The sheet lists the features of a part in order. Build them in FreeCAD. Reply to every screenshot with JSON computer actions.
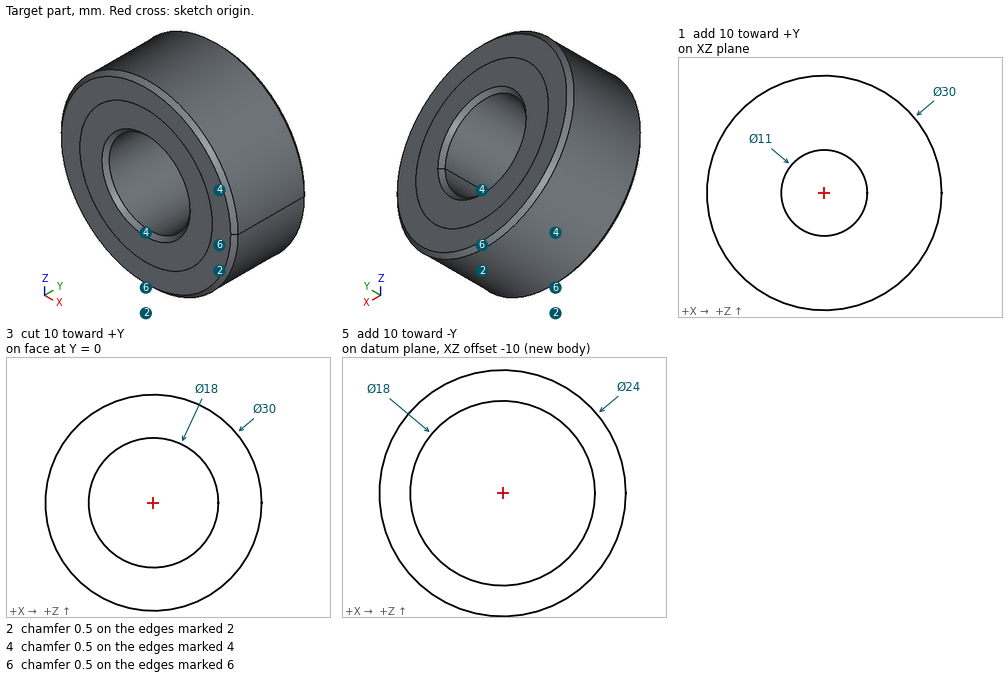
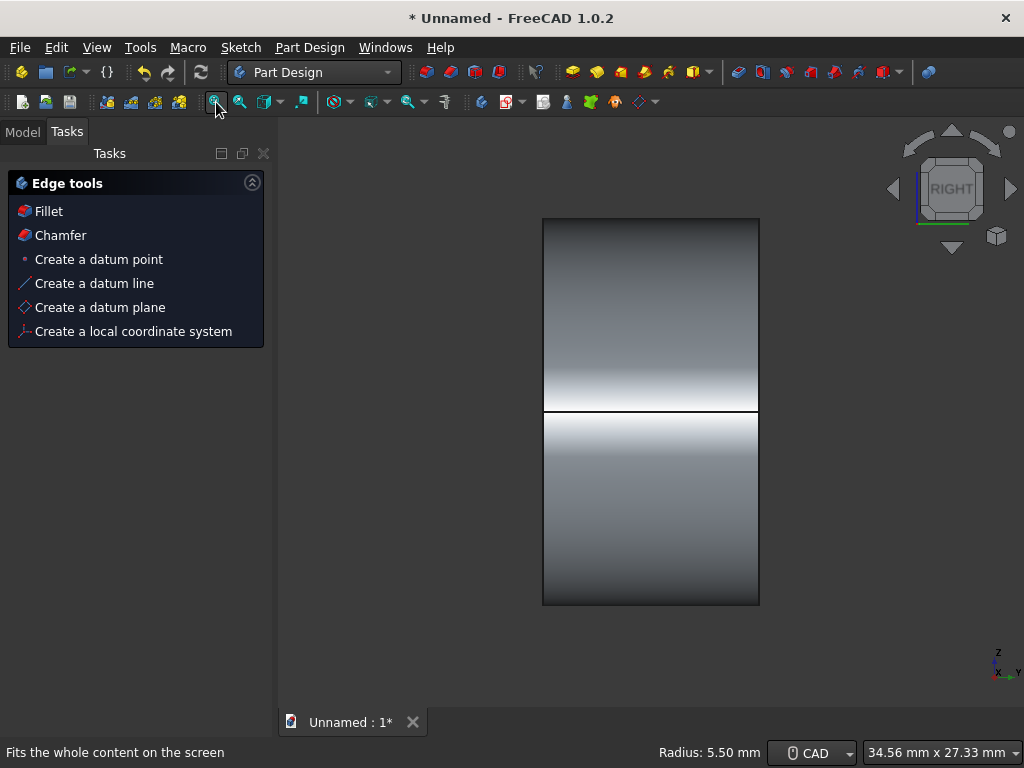
{"action": "key", "text": "5"}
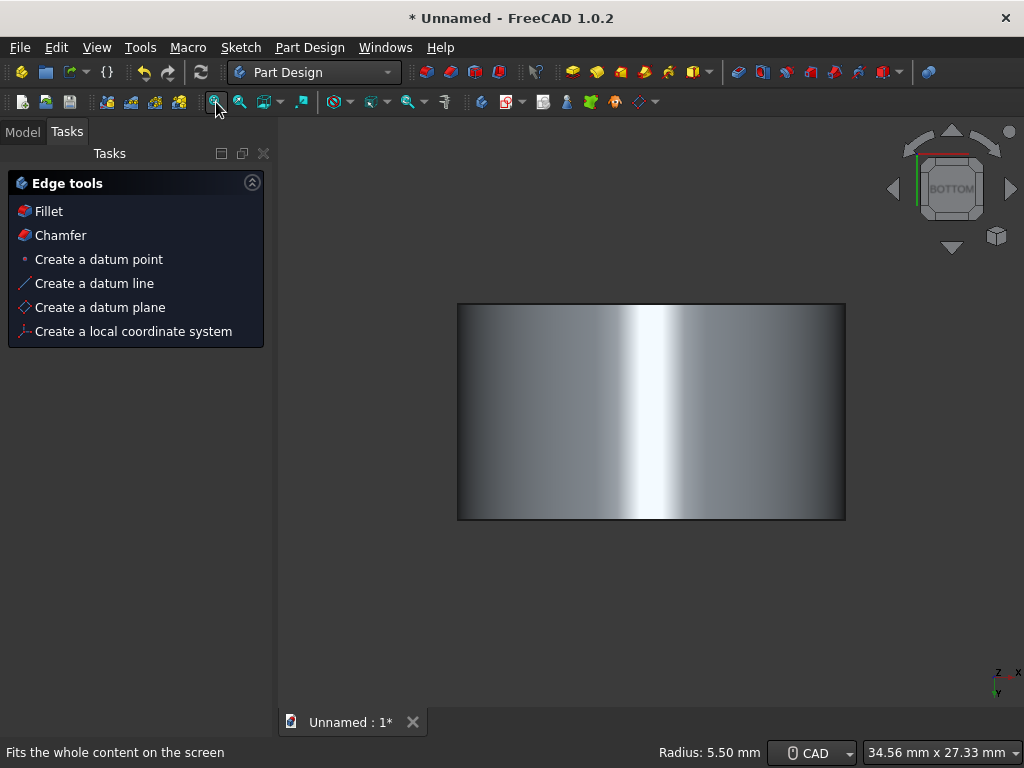
{"action": "key", "text": "4"}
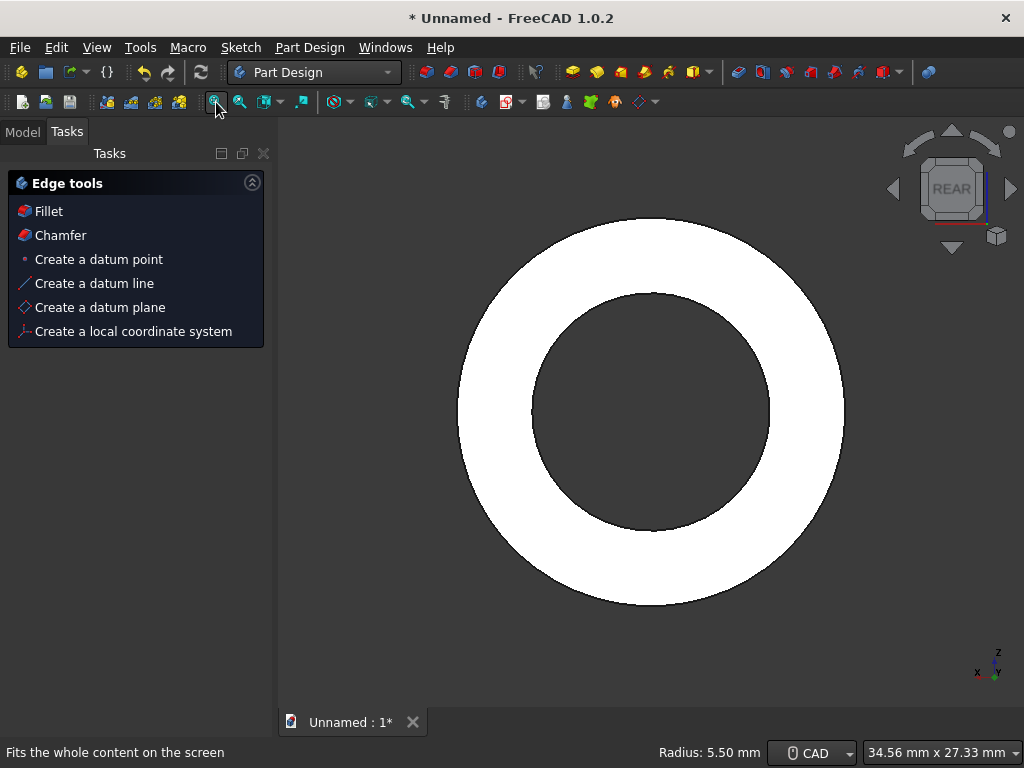
{"action": "left_click", "coordinate": [770, 411], "text": "ctrl"}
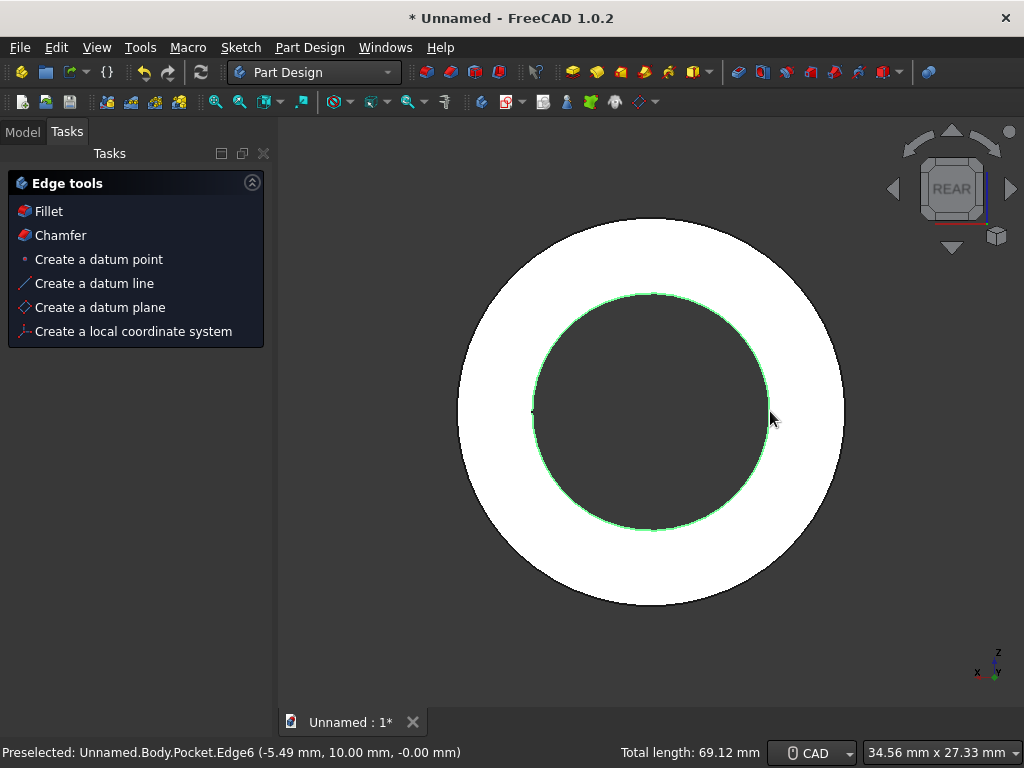
{"action": "left_click", "coordinate": [452, 72]}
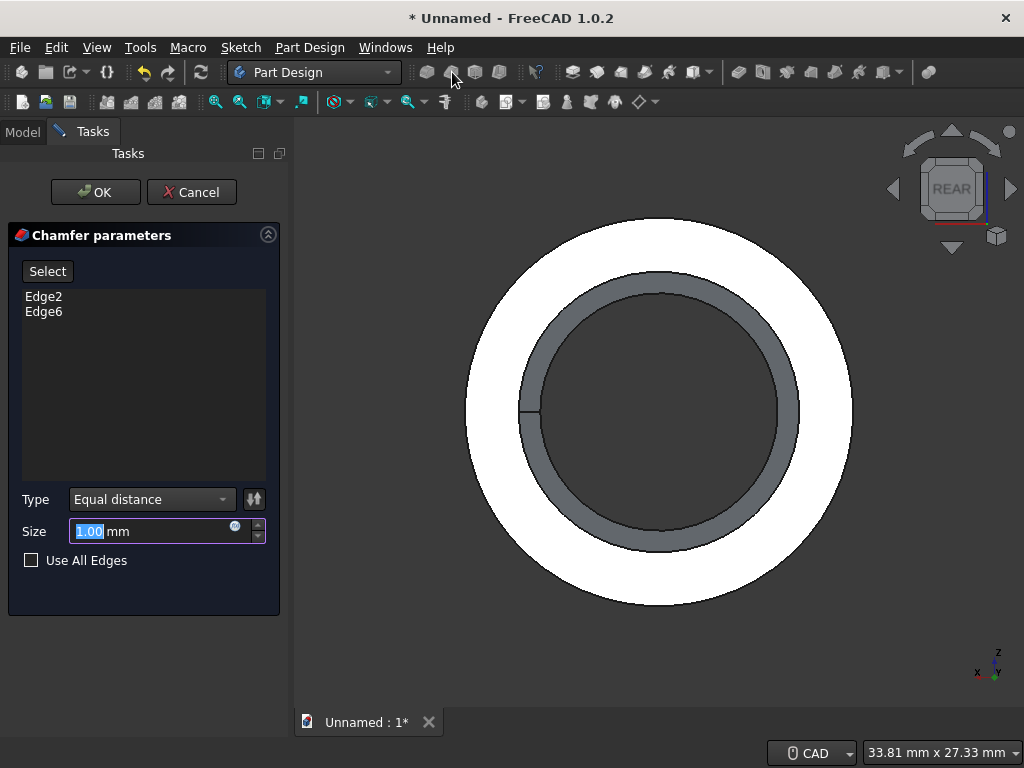
{"action": "type", "text": "0.5"}
{"action": "key", "text": "Tab"}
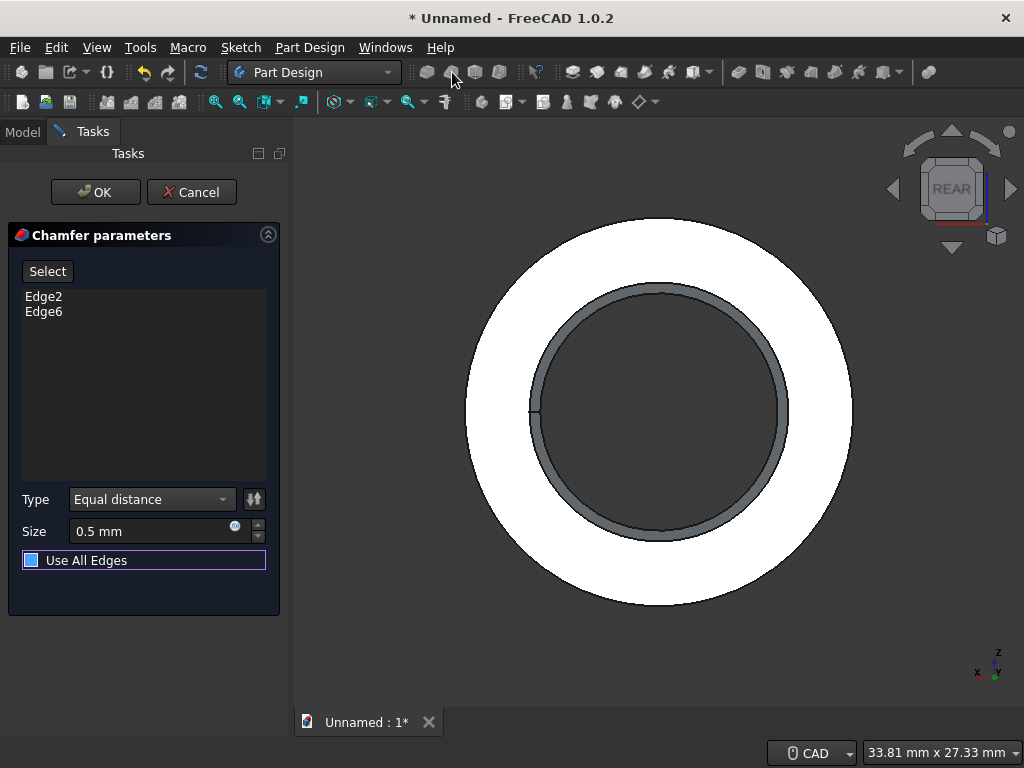
{"action": "left_click", "coordinate": [96, 192]}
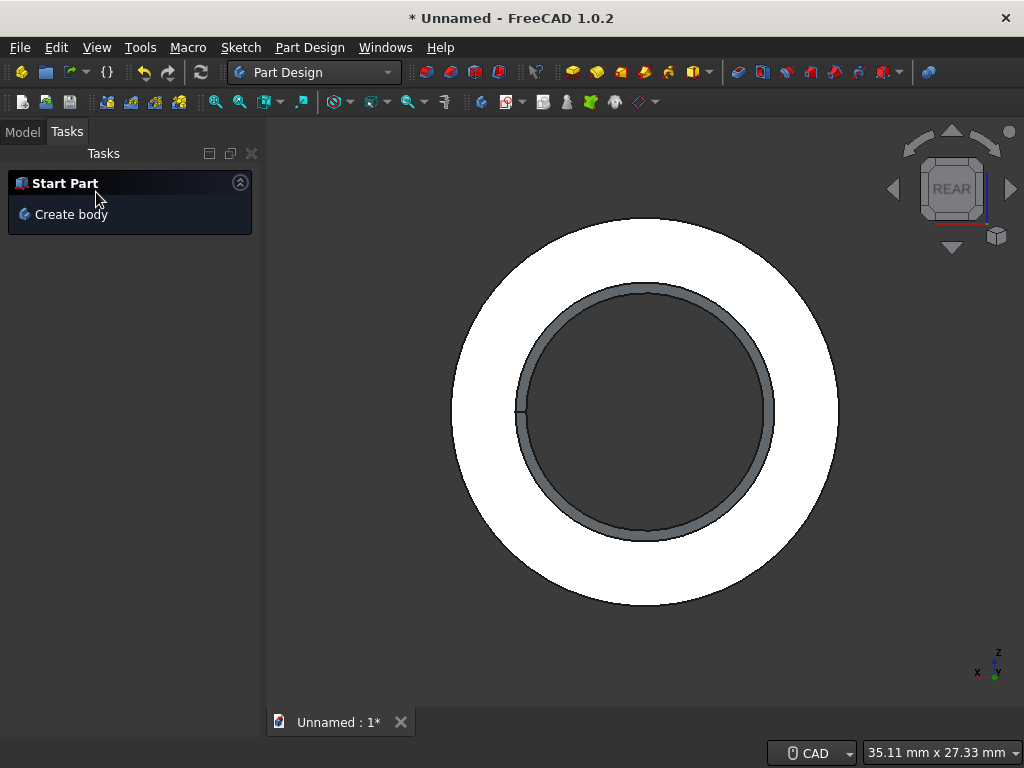
{"action": "left_click", "coordinate": [482, 102]}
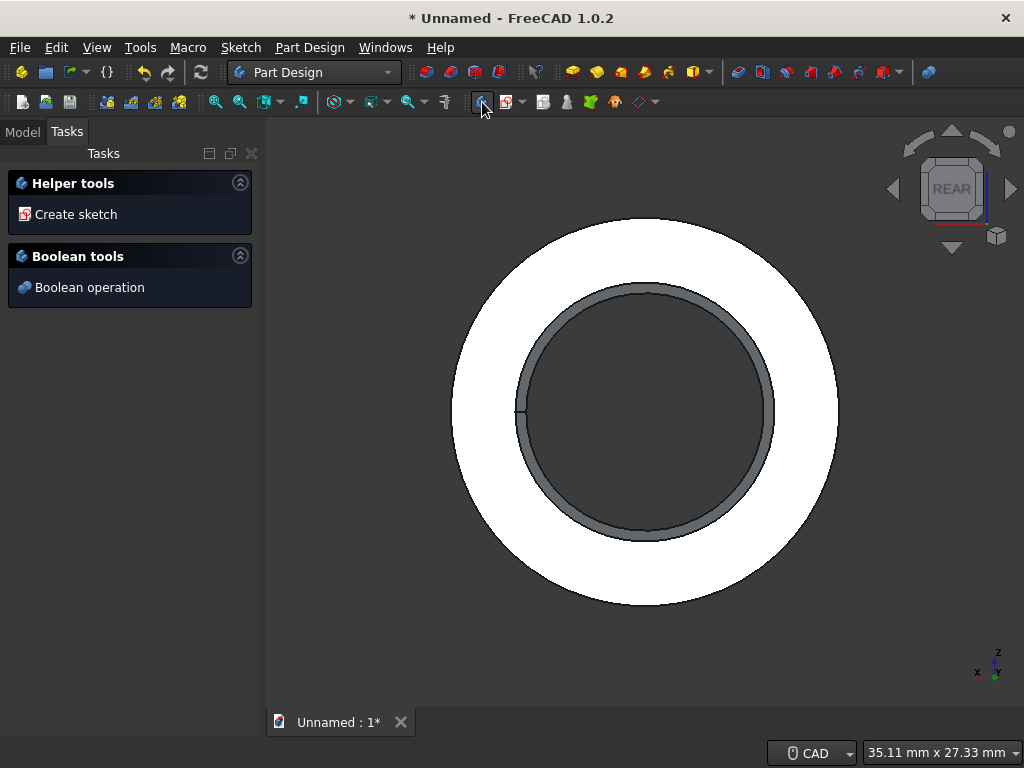
{"action": "left_click", "coordinate": [23, 131]}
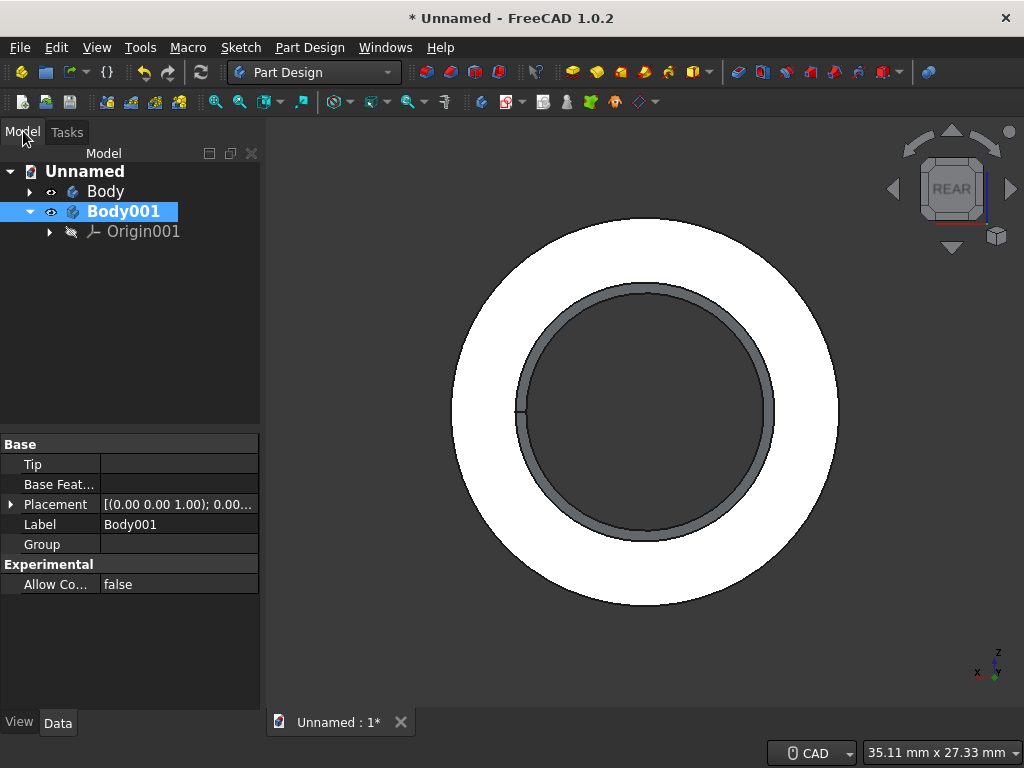
{"action": "left_click", "coordinate": [50, 232]}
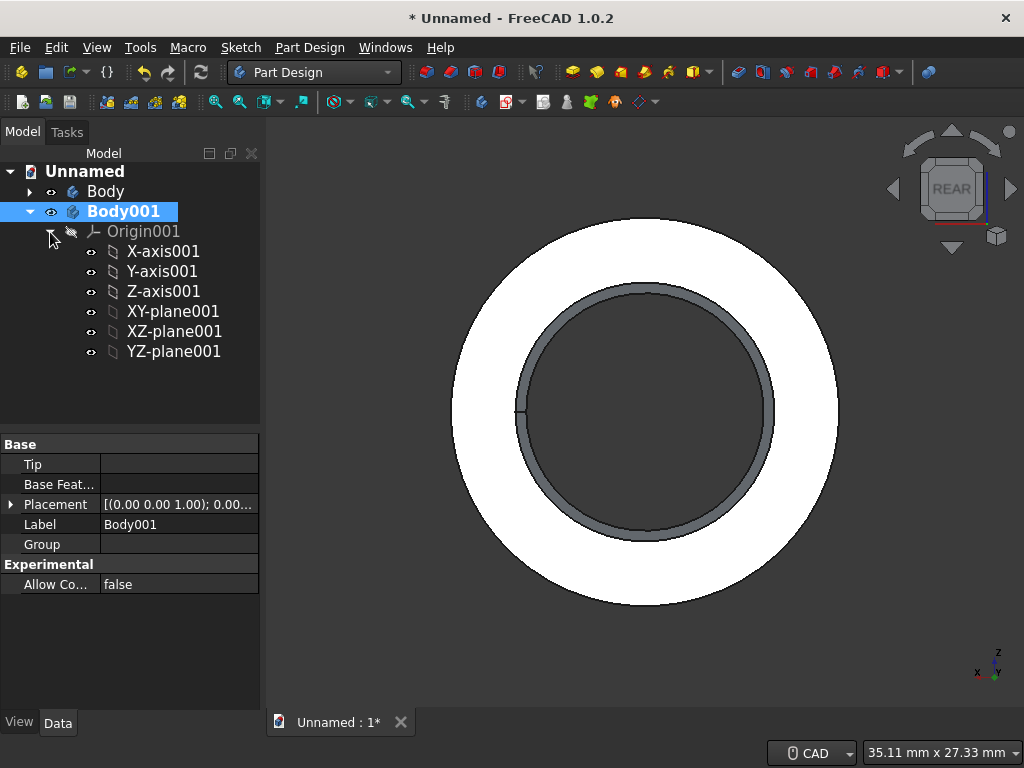
{"action": "left_click", "coordinate": [136, 332]}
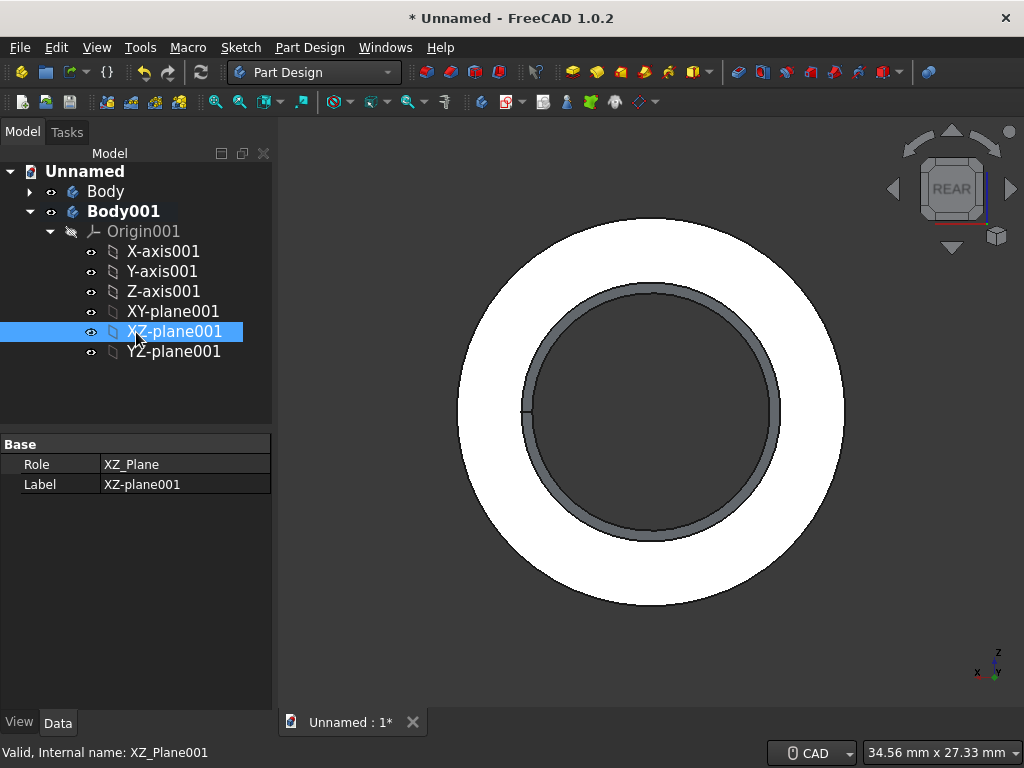
{"action": "left_click", "coordinate": [640, 102]}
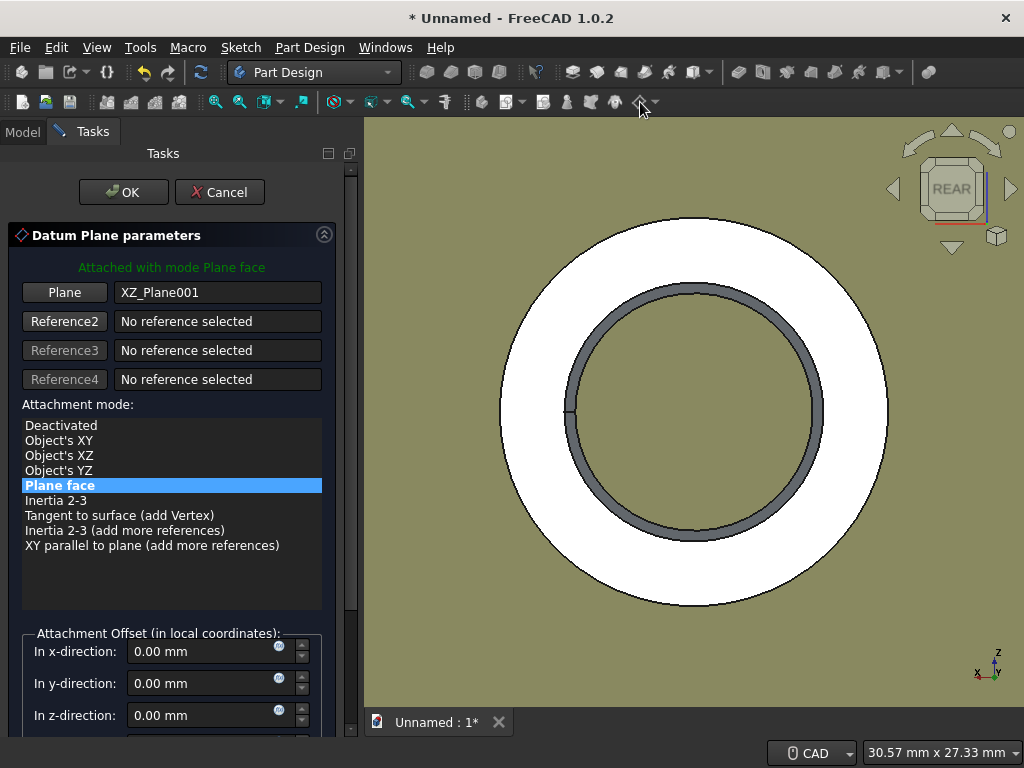
{"action": "triple_click", "coordinate": [210, 715]}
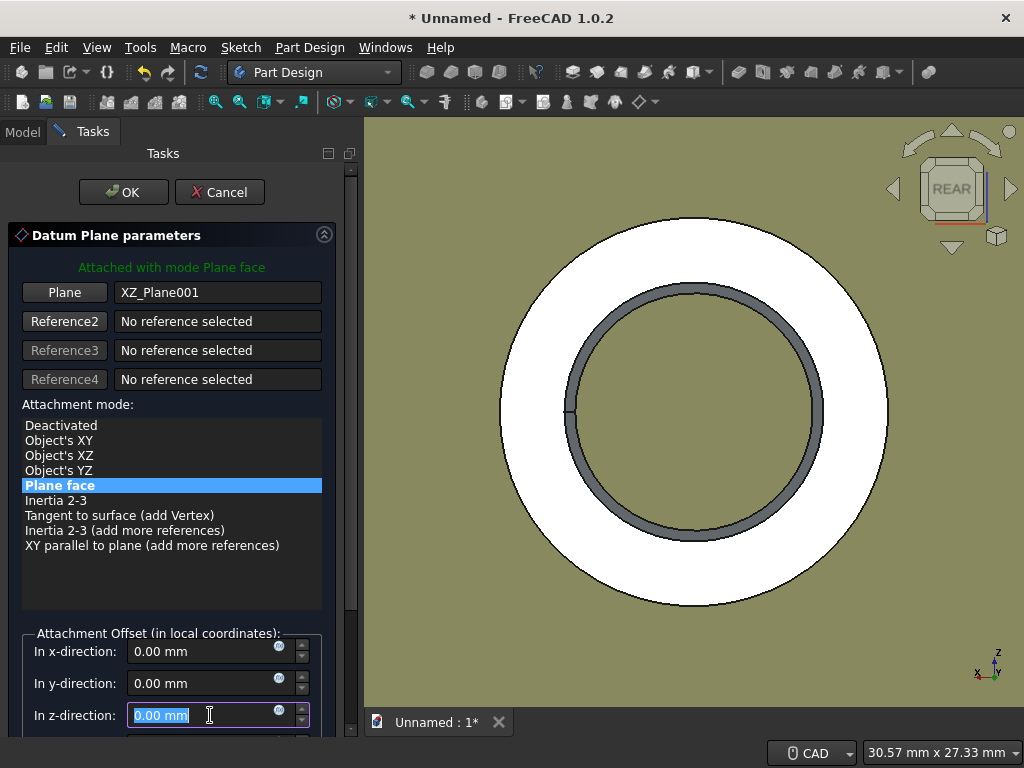
{"action": "type", "text": "-10"}
{"action": "key", "text": "Tab"}